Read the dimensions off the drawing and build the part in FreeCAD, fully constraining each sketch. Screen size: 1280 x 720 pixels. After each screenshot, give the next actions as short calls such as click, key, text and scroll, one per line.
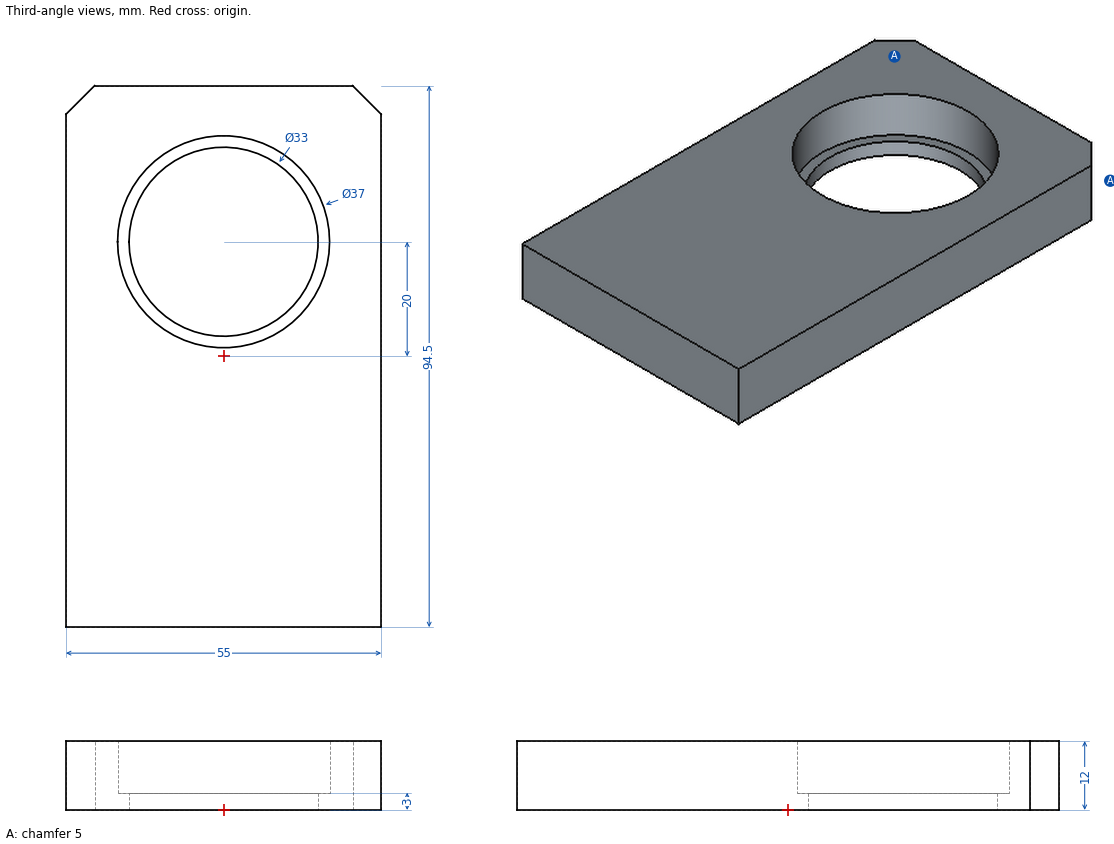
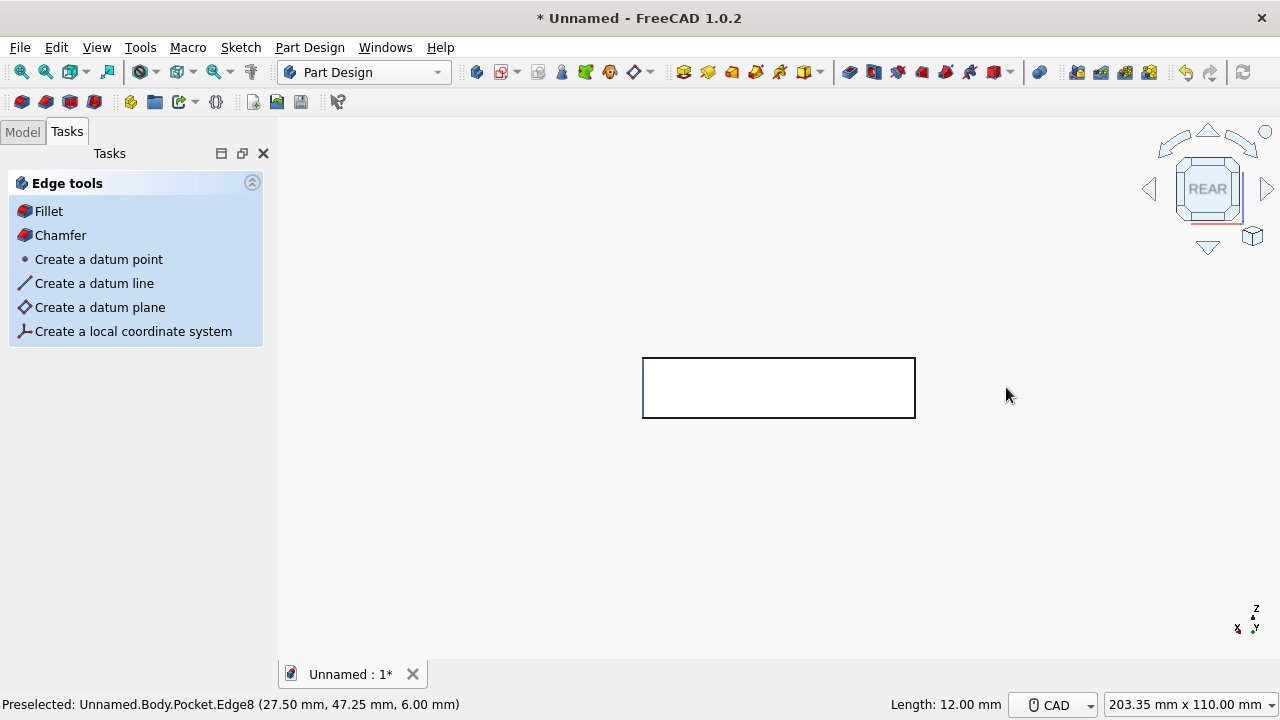
click(22, 72)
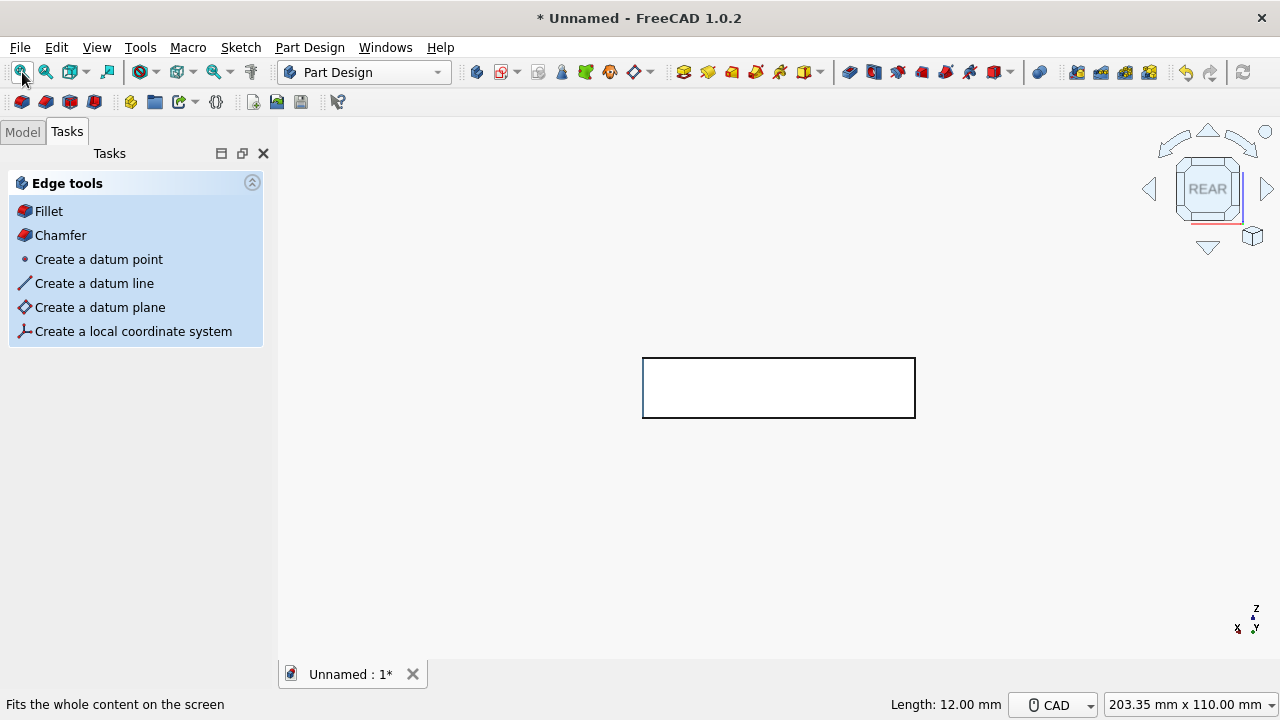
click(915, 387, ctrl)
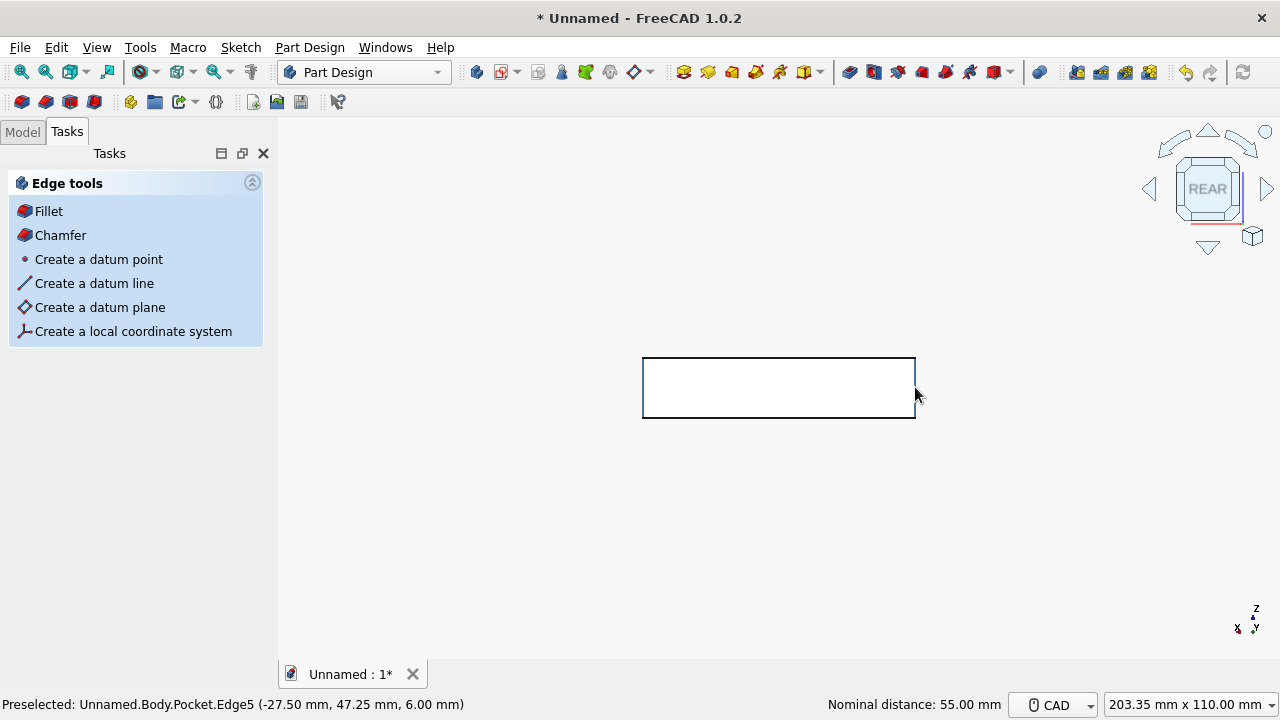
click(46, 102)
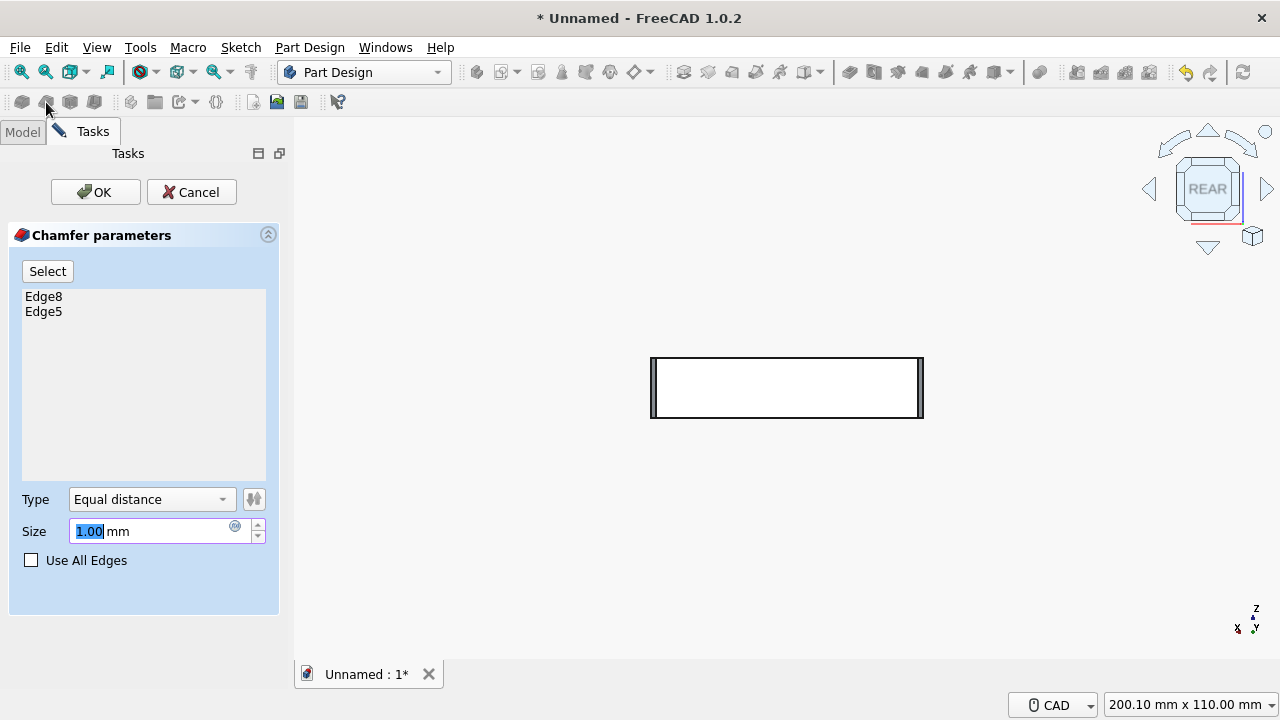
text(5)
key(Tab)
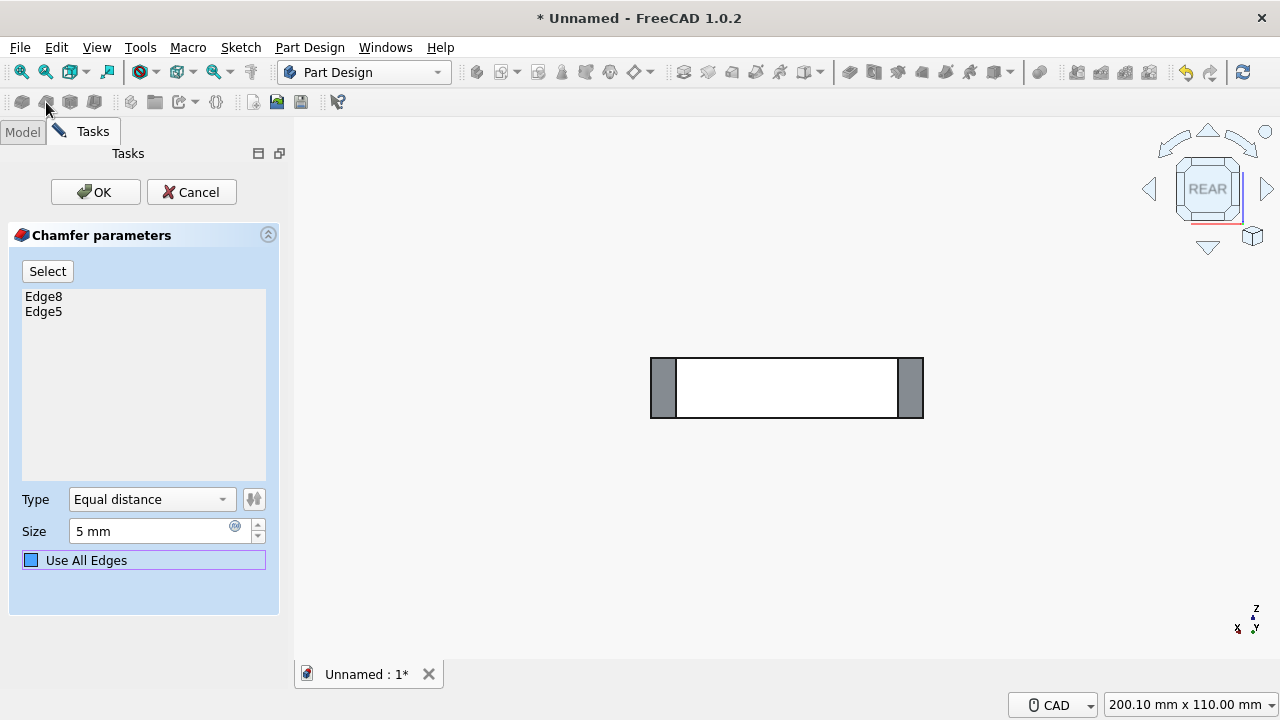
click(96, 192)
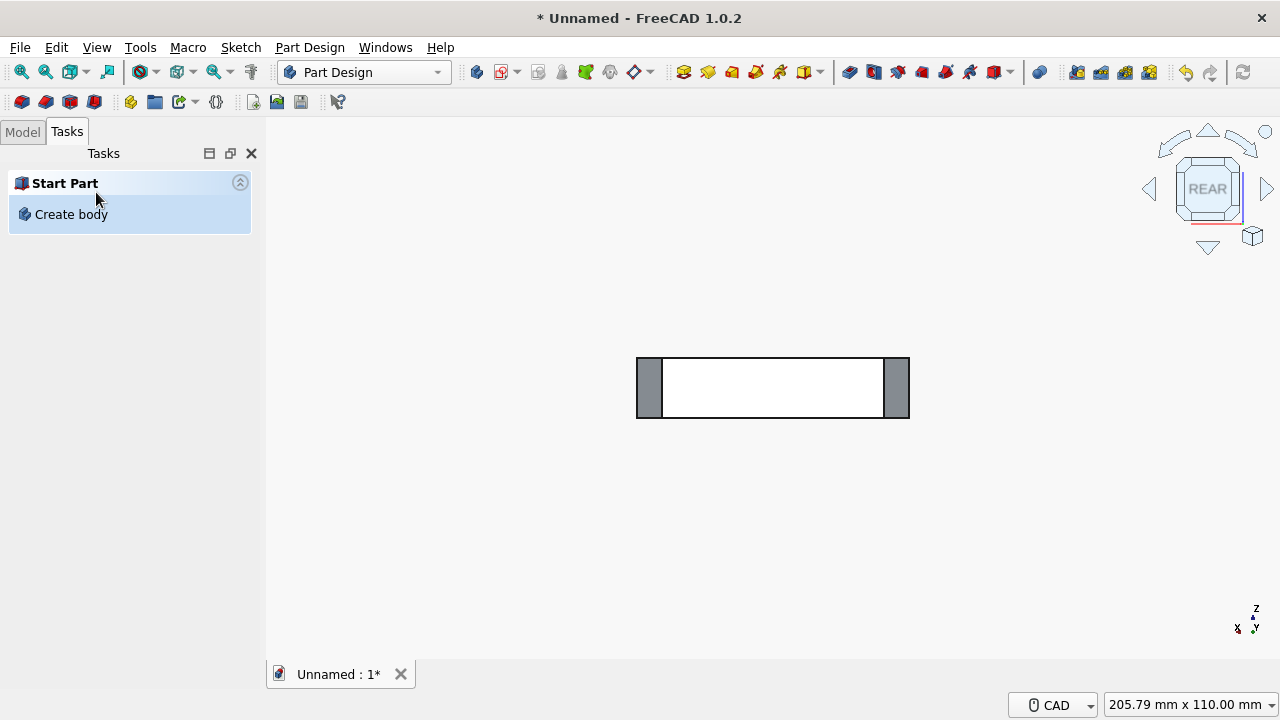
click(22, 72)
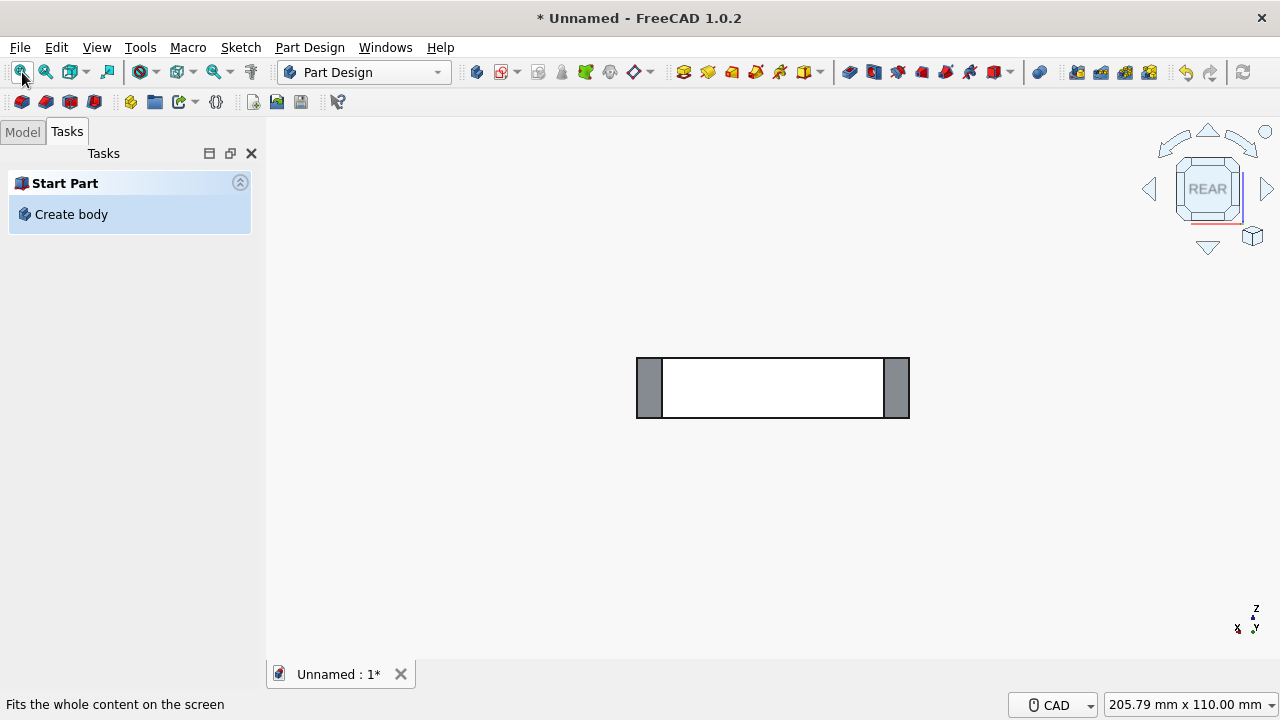
click(502, 72)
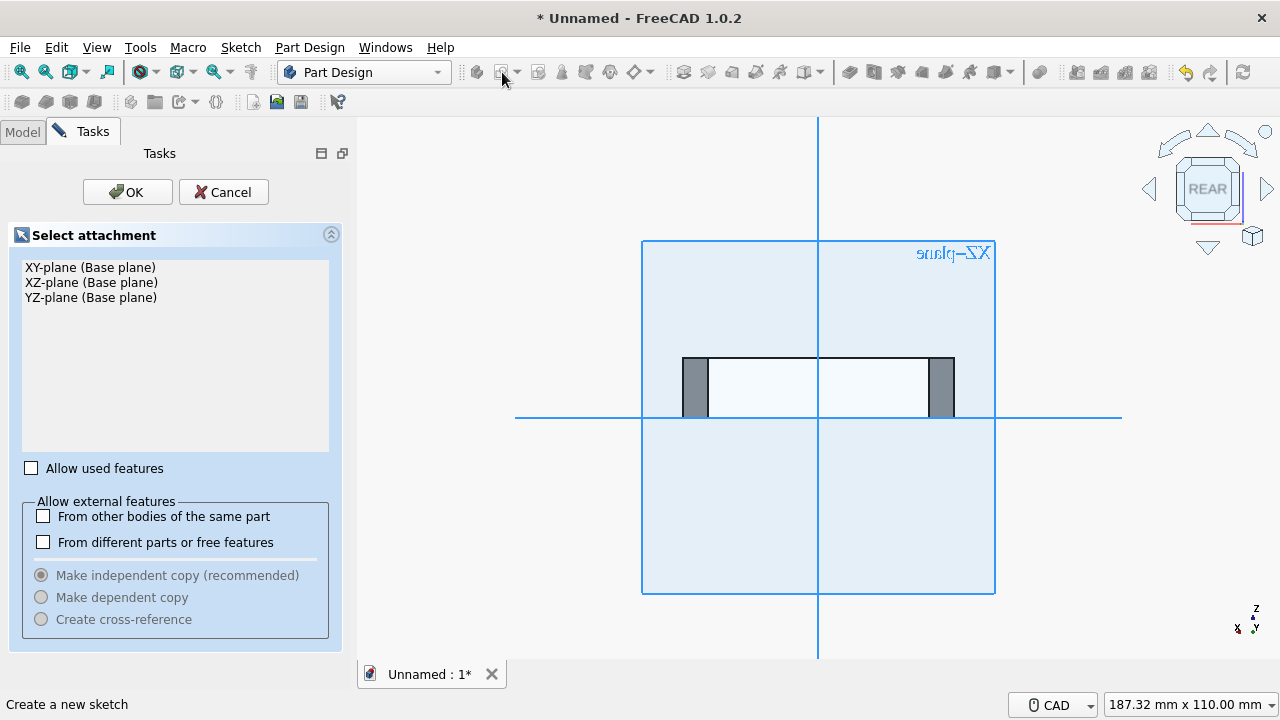
click(82, 268)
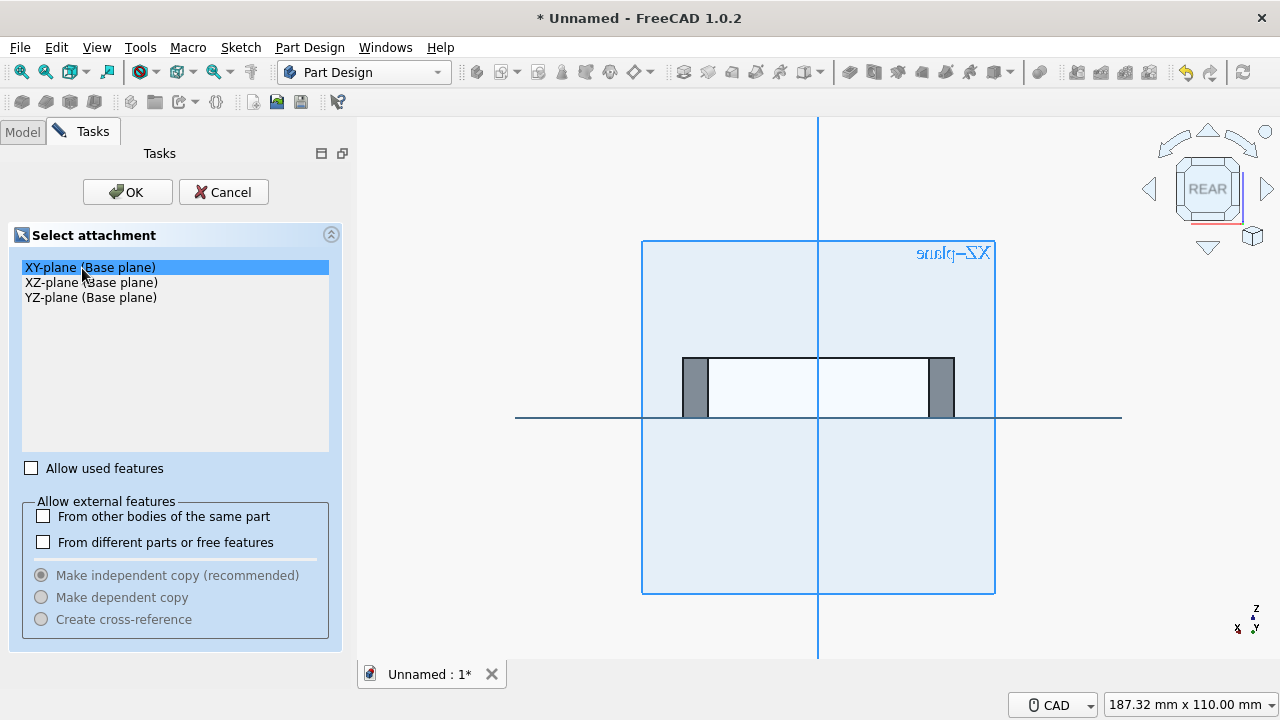
click(128, 192)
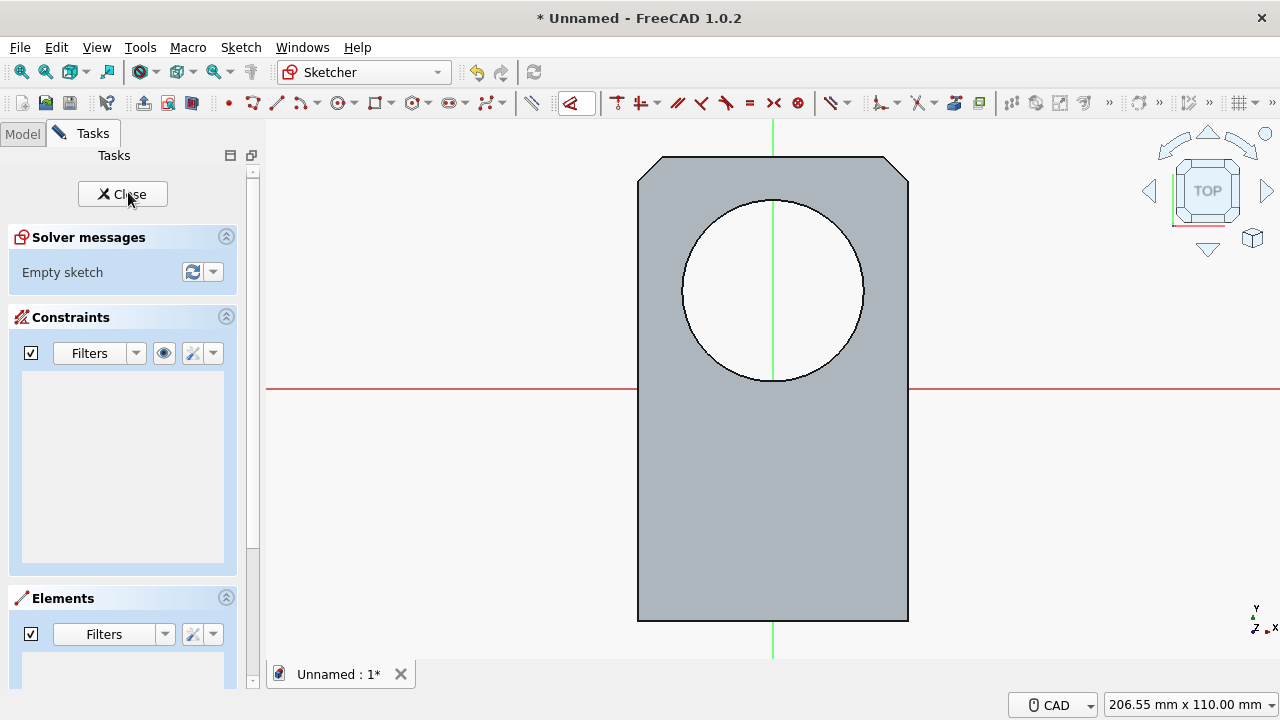
click(192, 104)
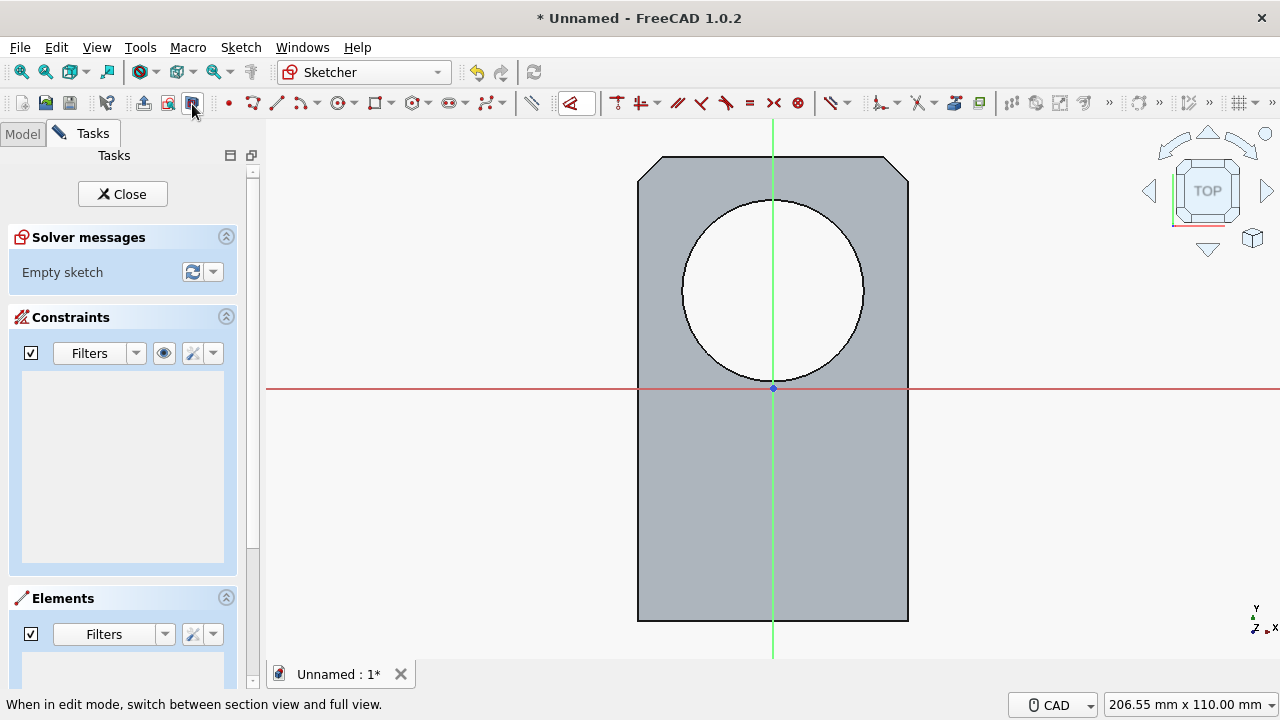
scroll(856, 180, up, 3)